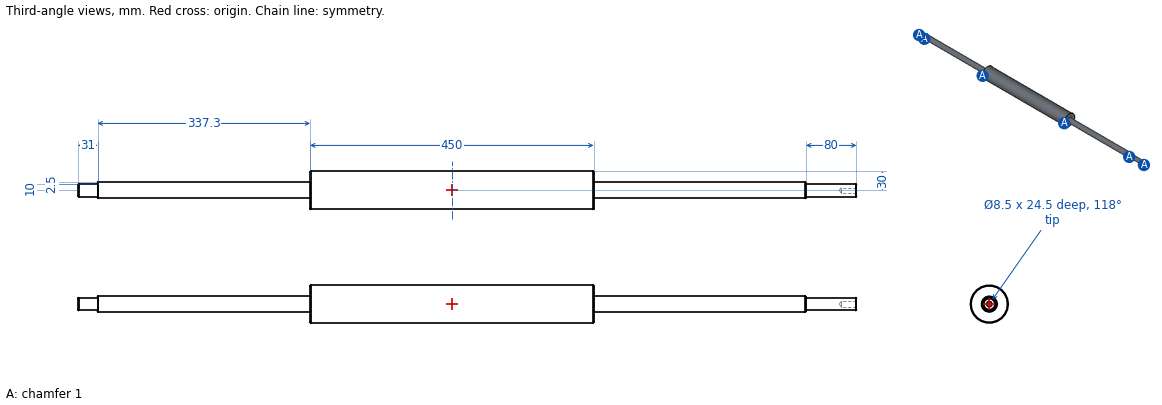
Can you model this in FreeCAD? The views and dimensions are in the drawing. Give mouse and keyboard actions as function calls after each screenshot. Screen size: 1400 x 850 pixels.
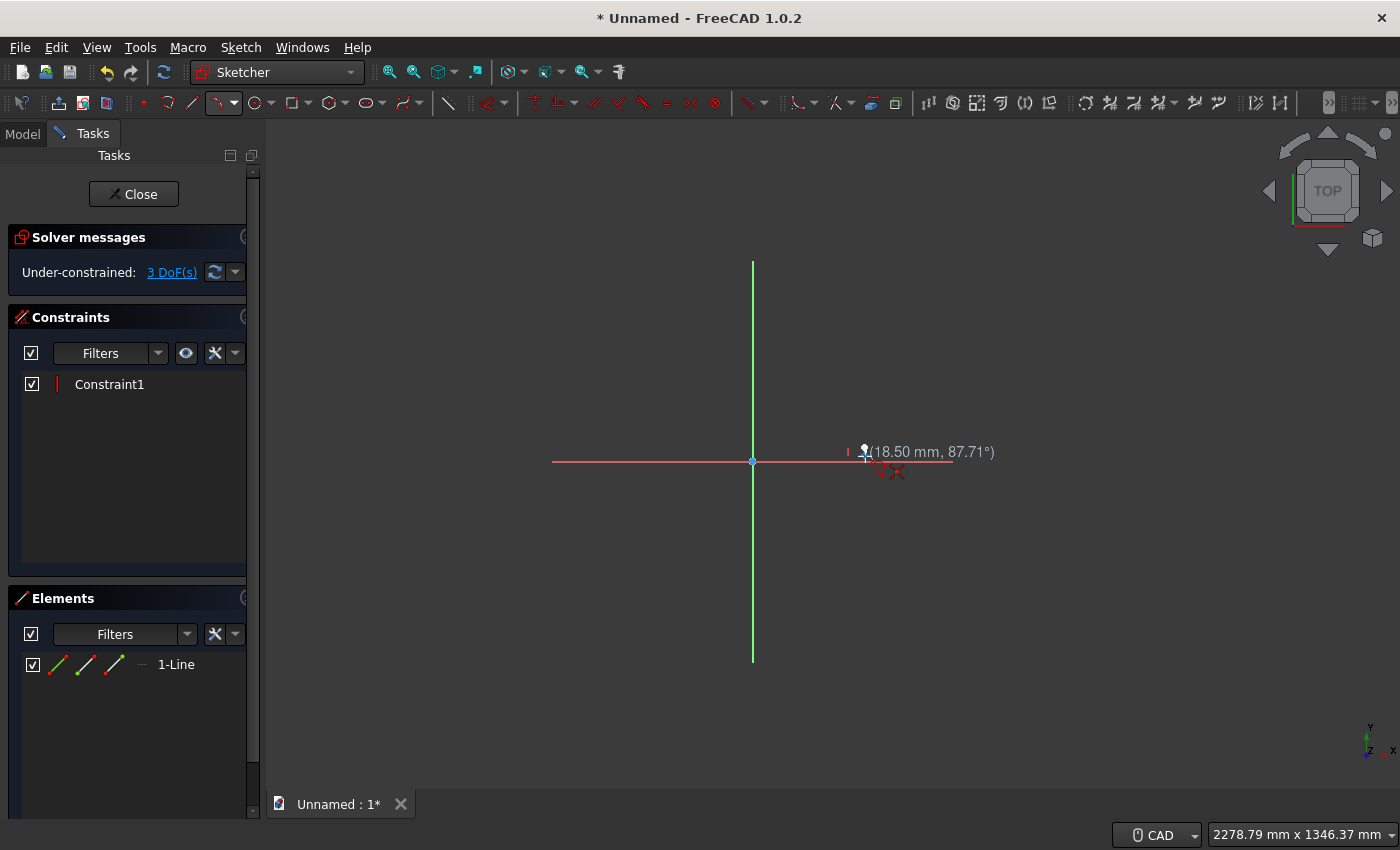
click(641, 447)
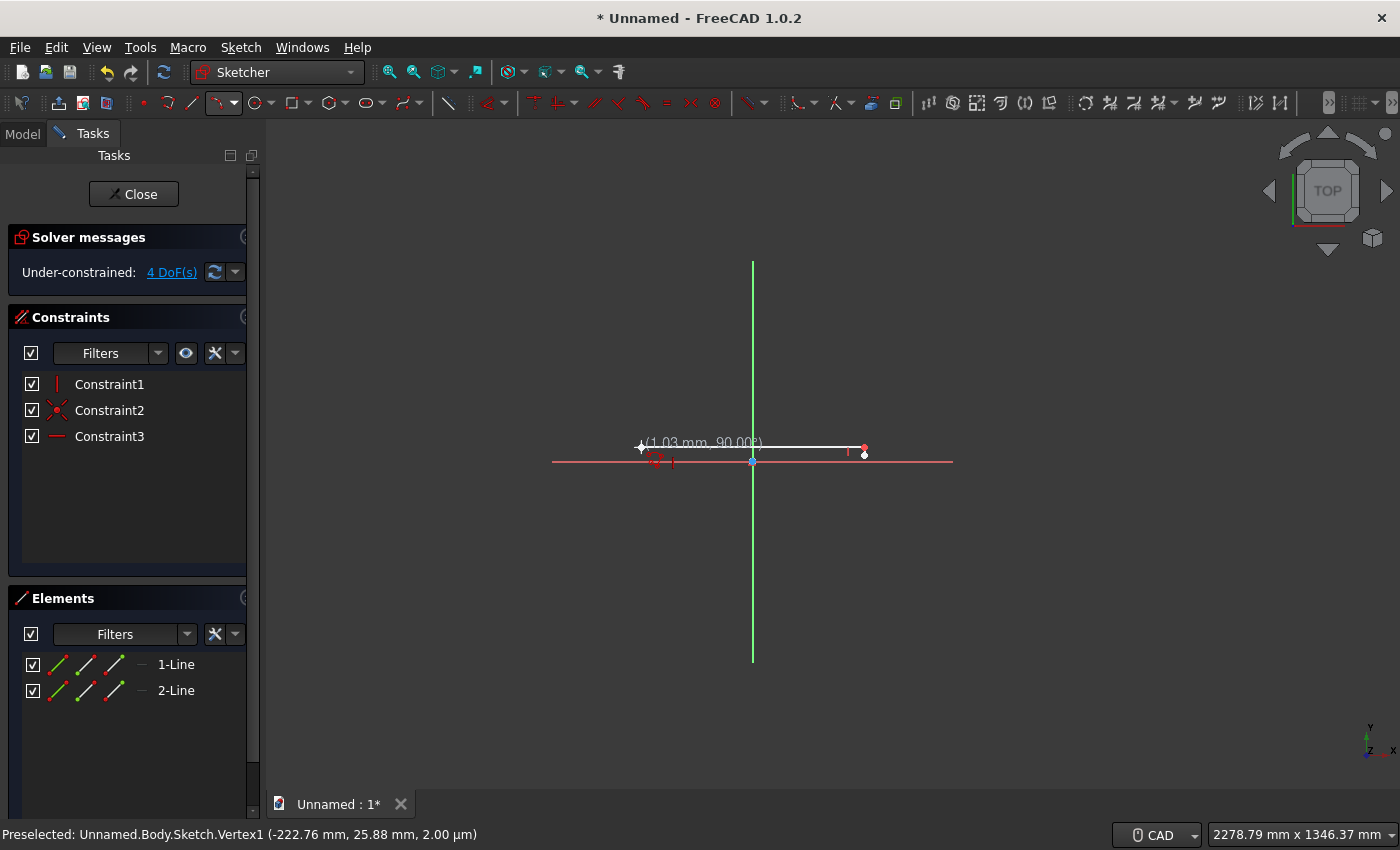
scroll(641, 456, up, 5)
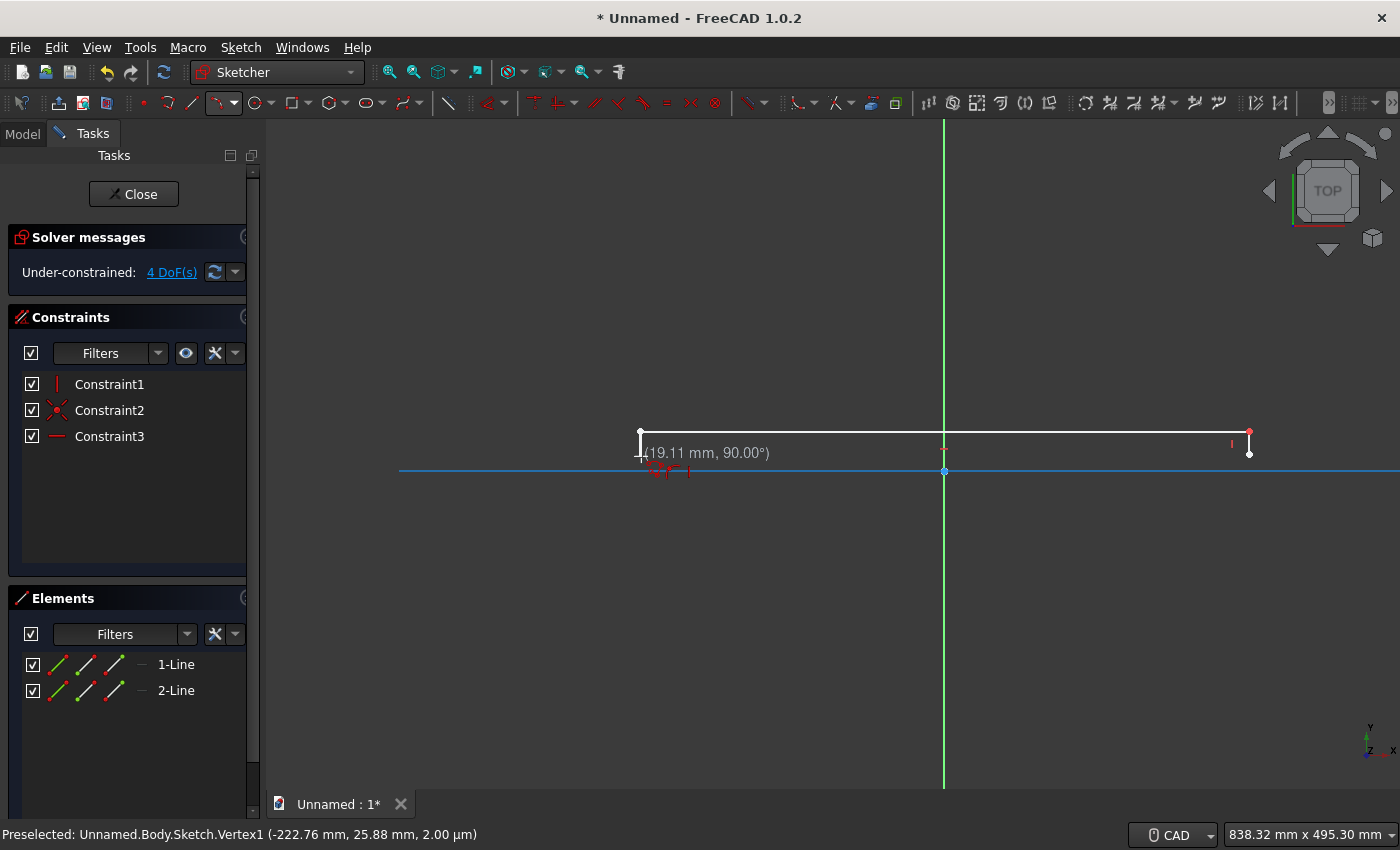
click(640, 454)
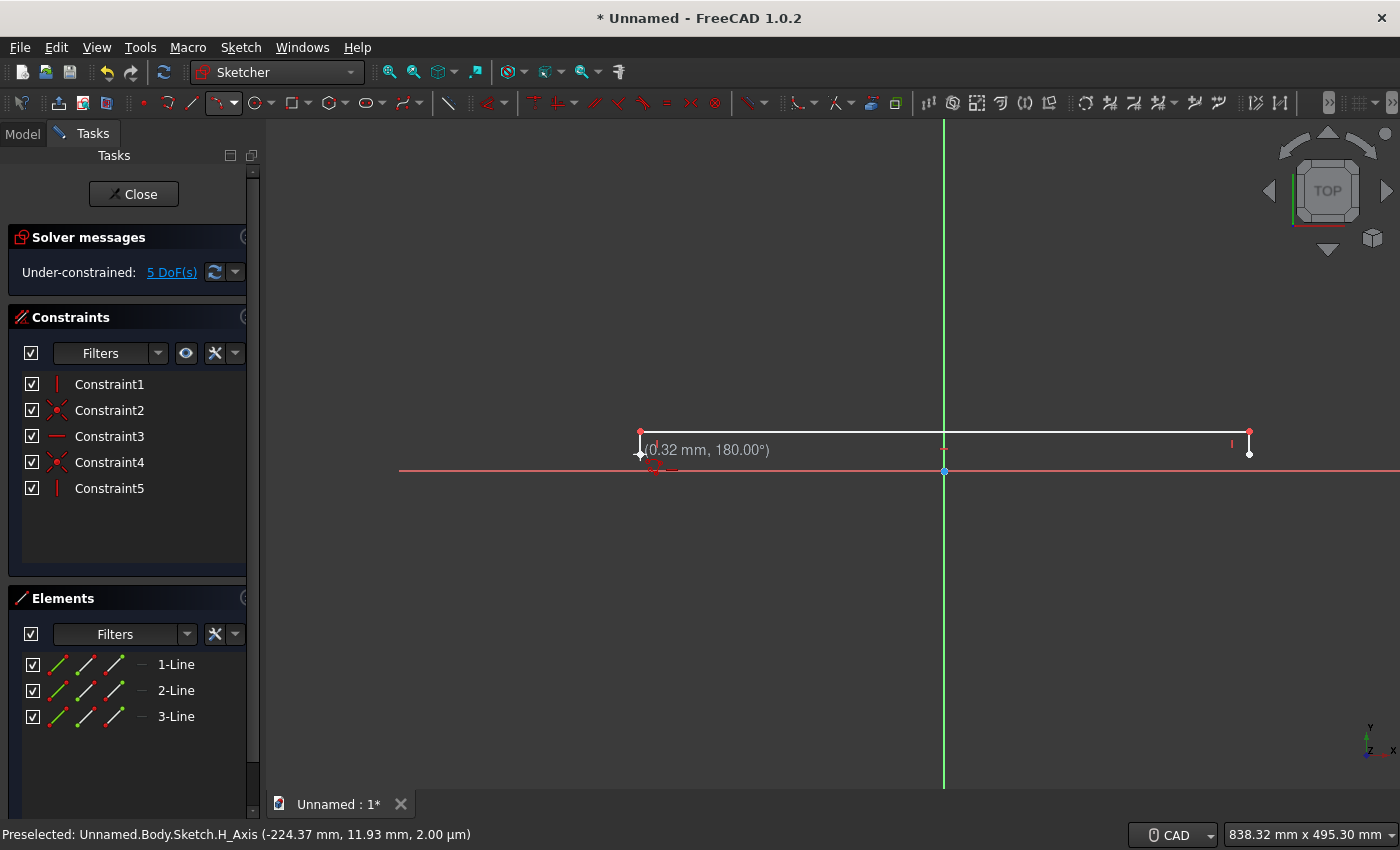
scroll(640, 456, down, 5)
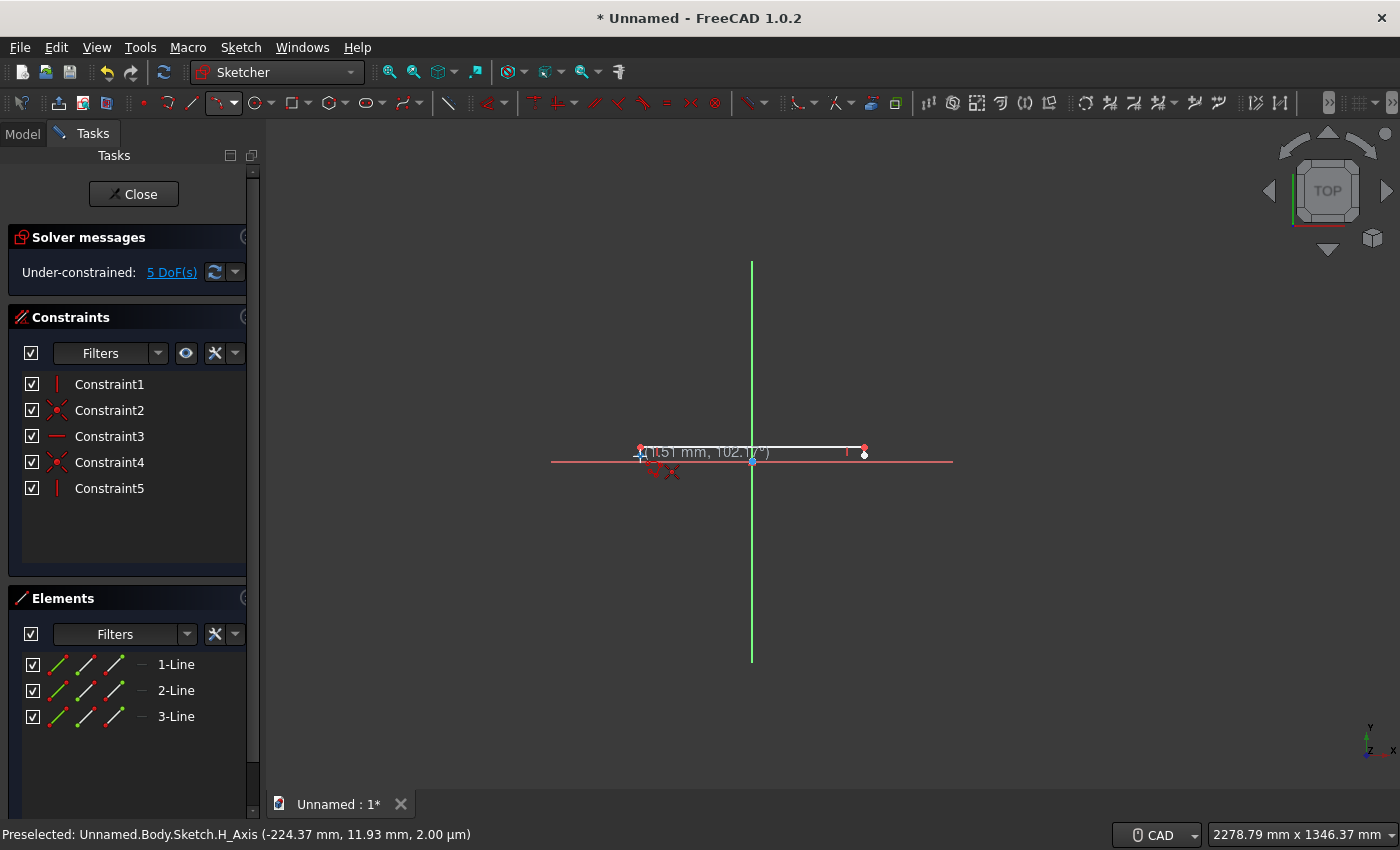
scroll(472, 456, up, 5)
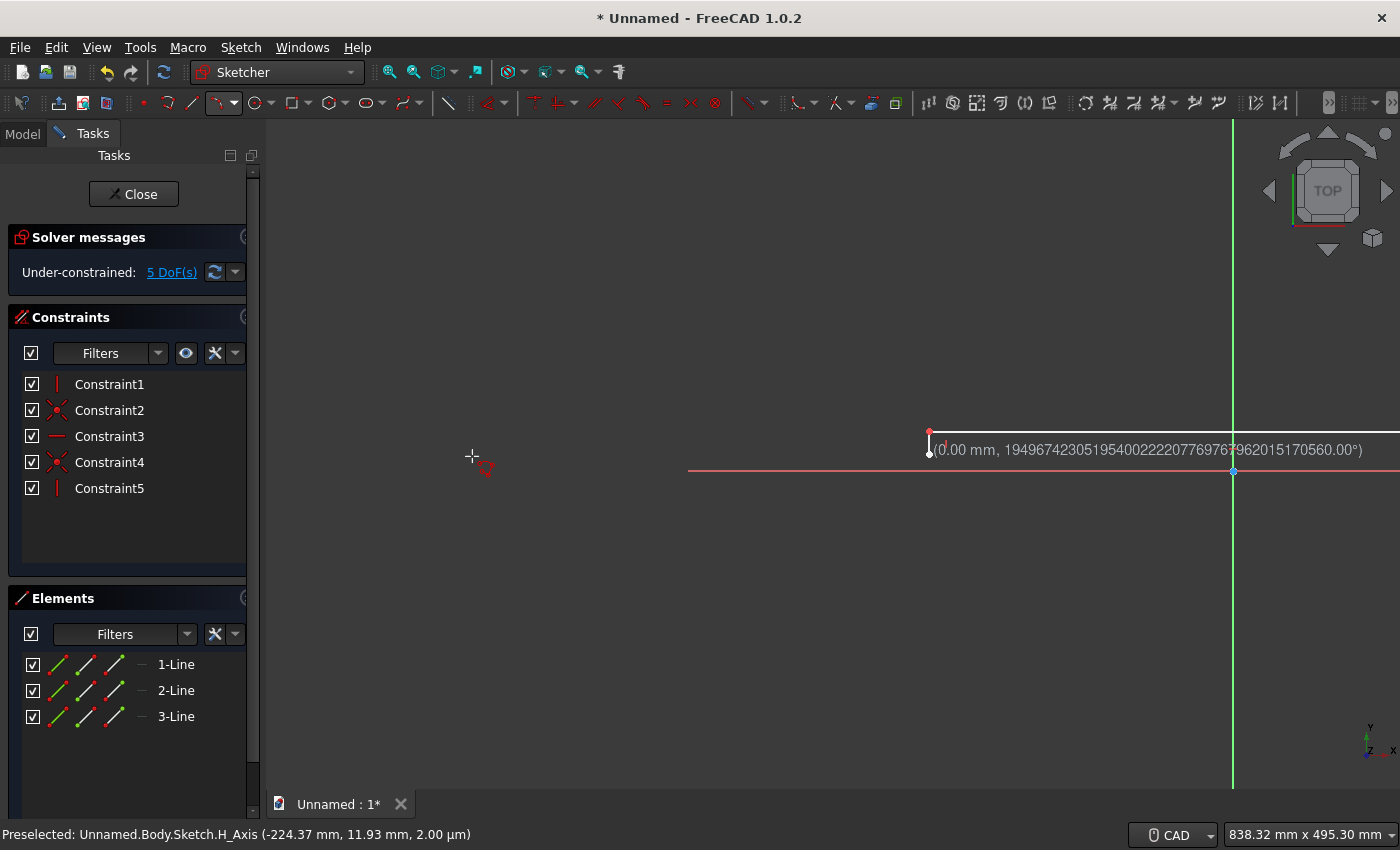
click(473, 454)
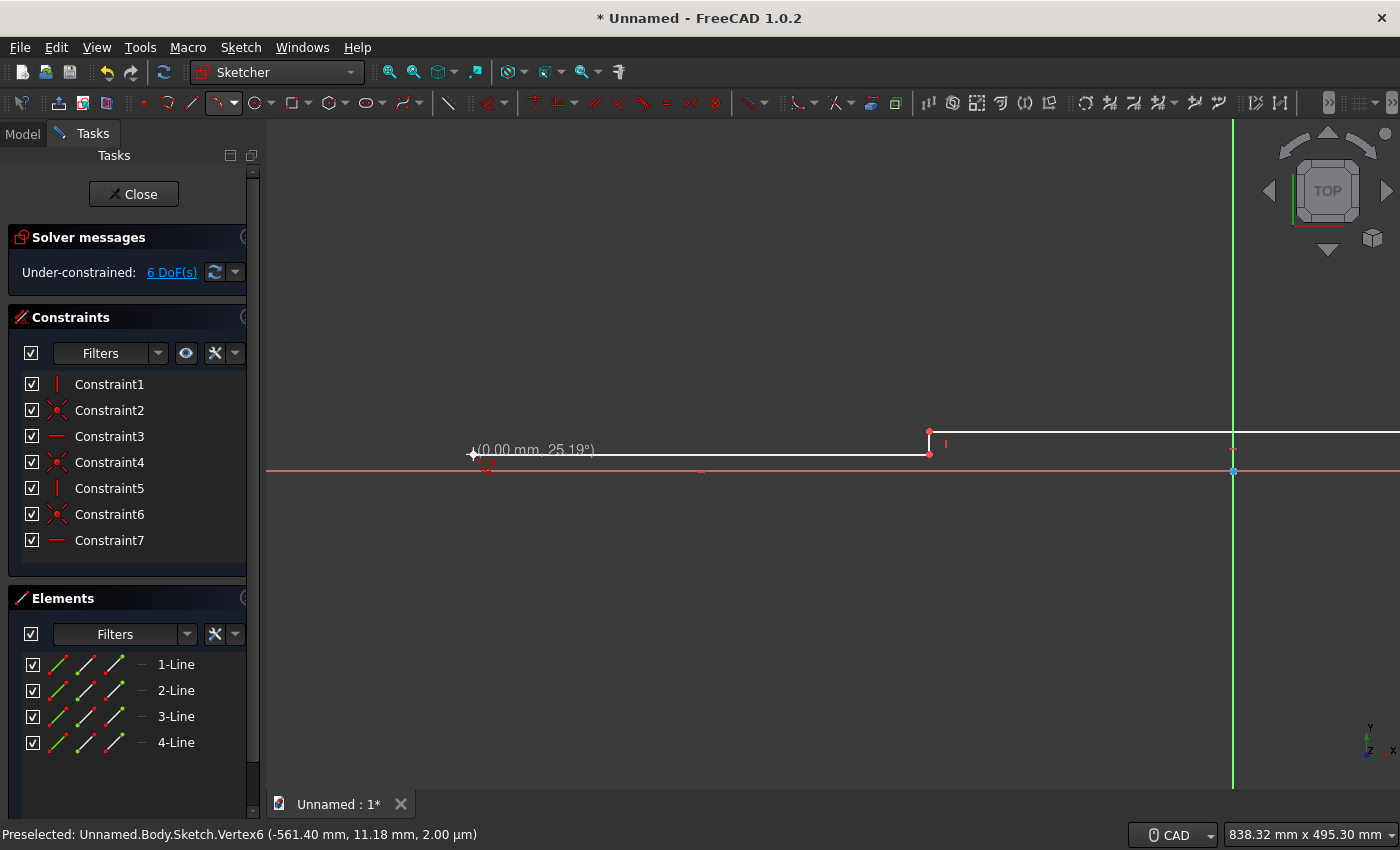
scroll(473, 458, up, 8)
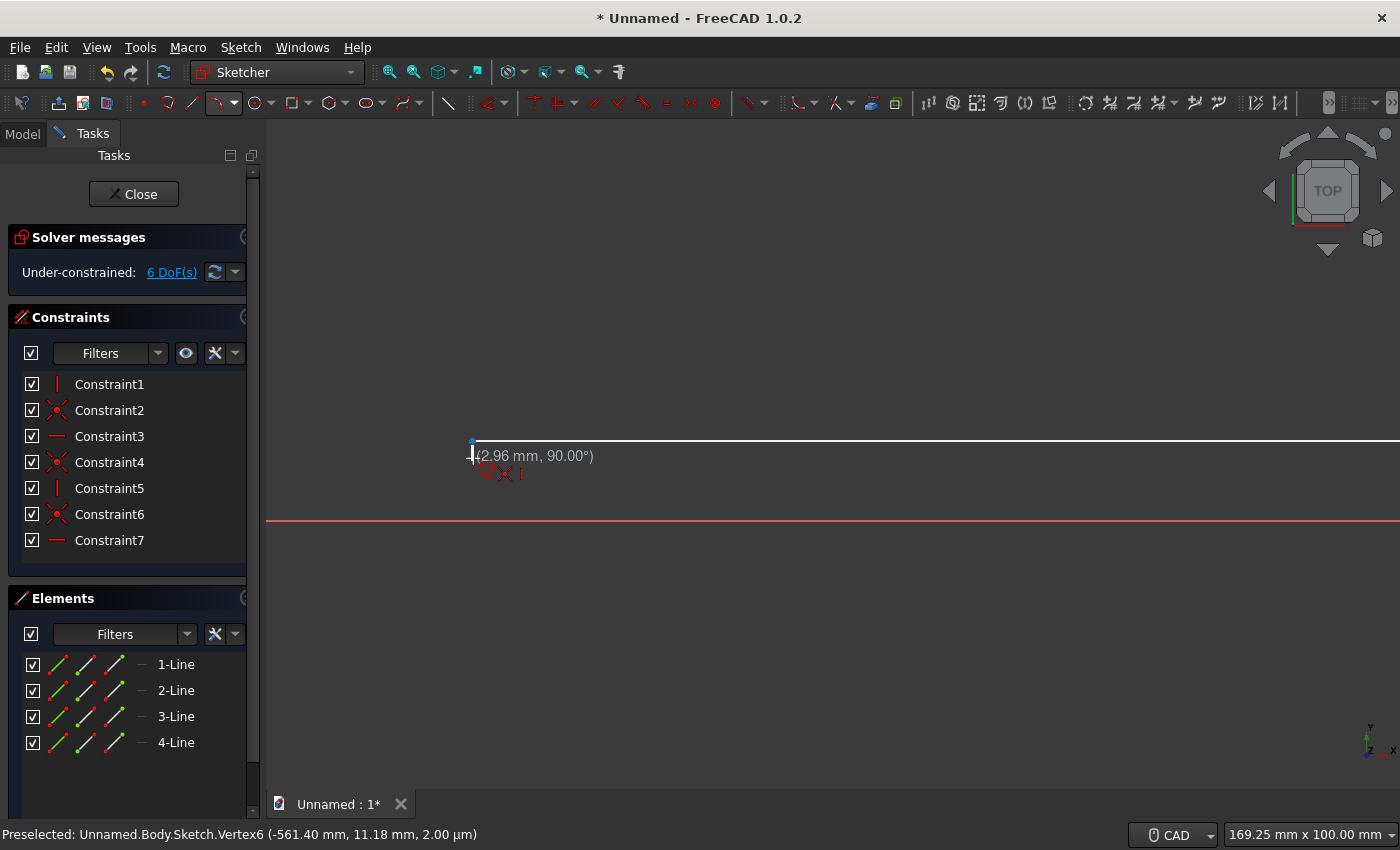
click(472, 454)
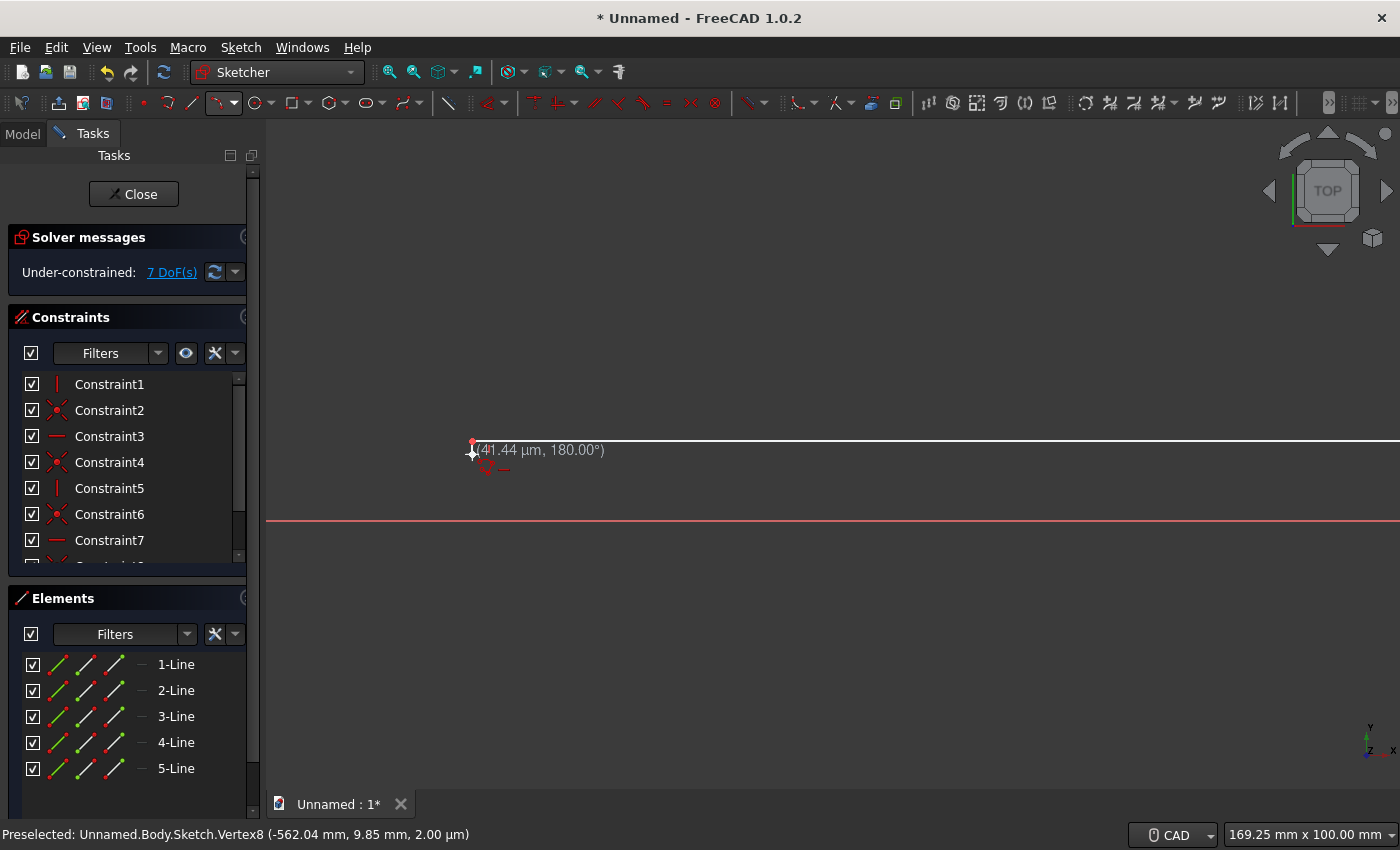
scroll(473, 457, down, 13)